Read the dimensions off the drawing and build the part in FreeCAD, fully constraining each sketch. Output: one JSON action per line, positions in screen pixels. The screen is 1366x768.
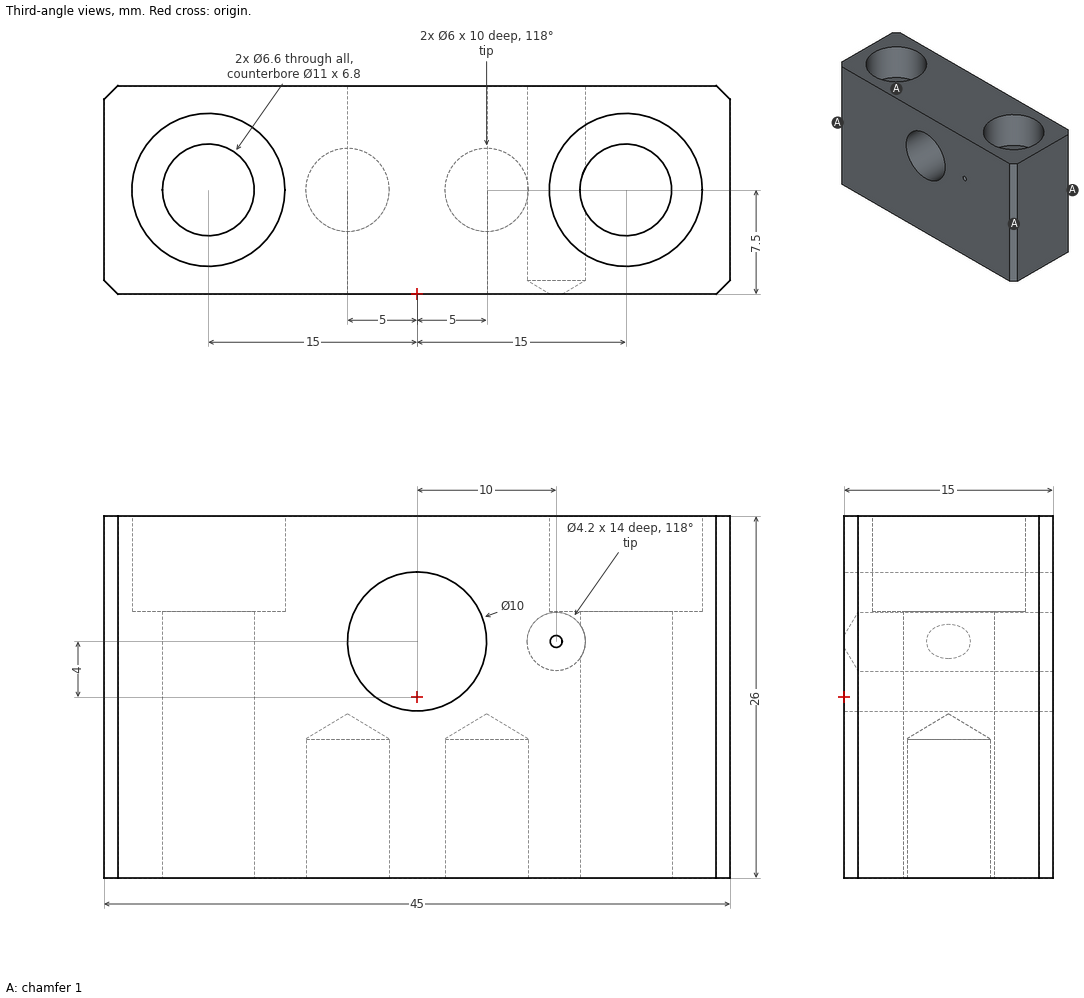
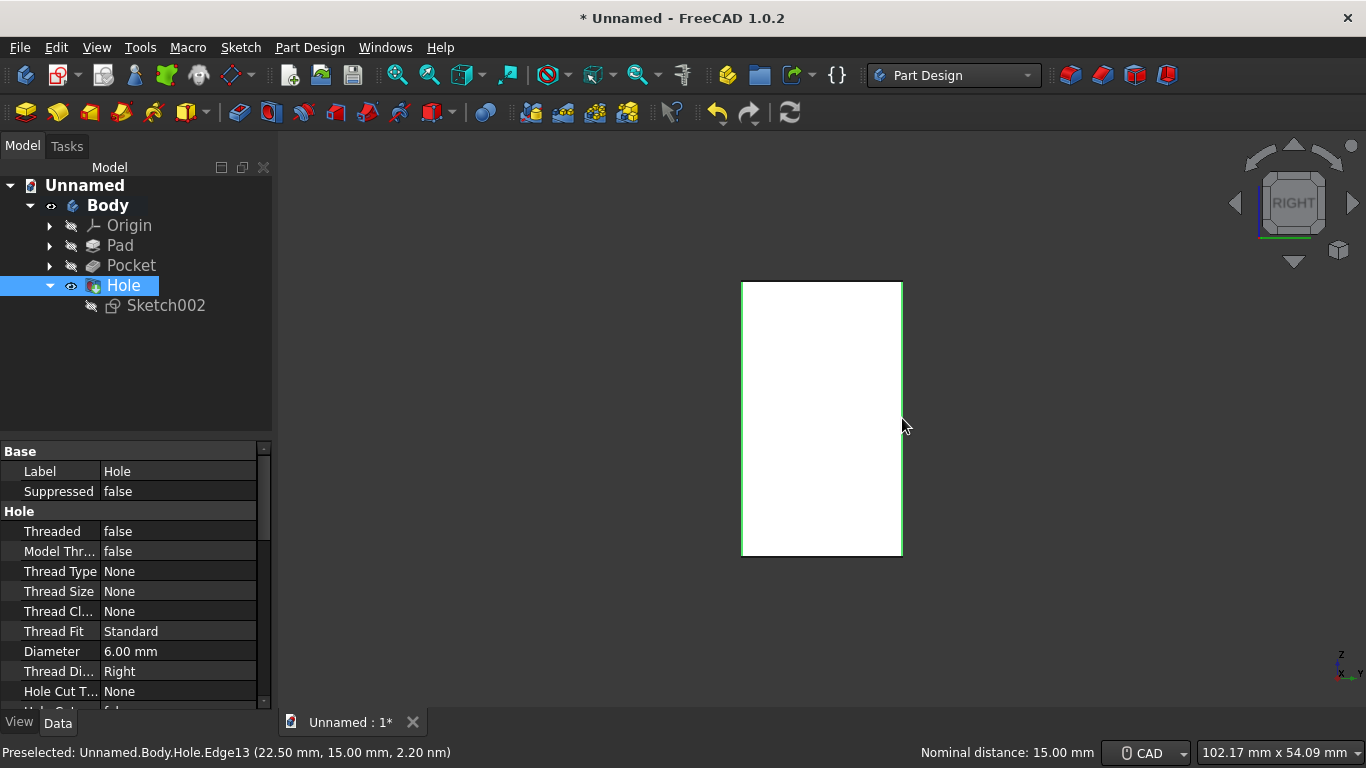
{"action": "key", "text": "5"}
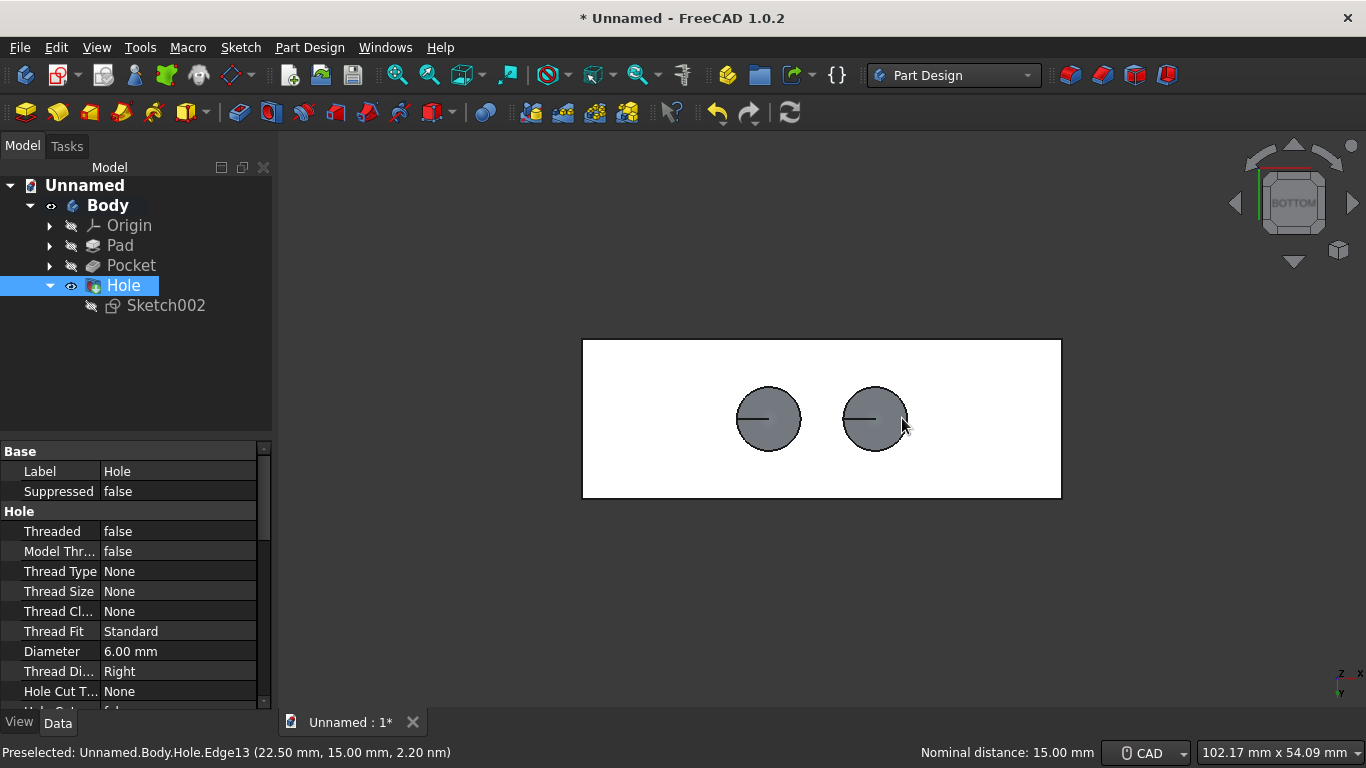
{"action": "left_click", "coordinate": [398, 76]}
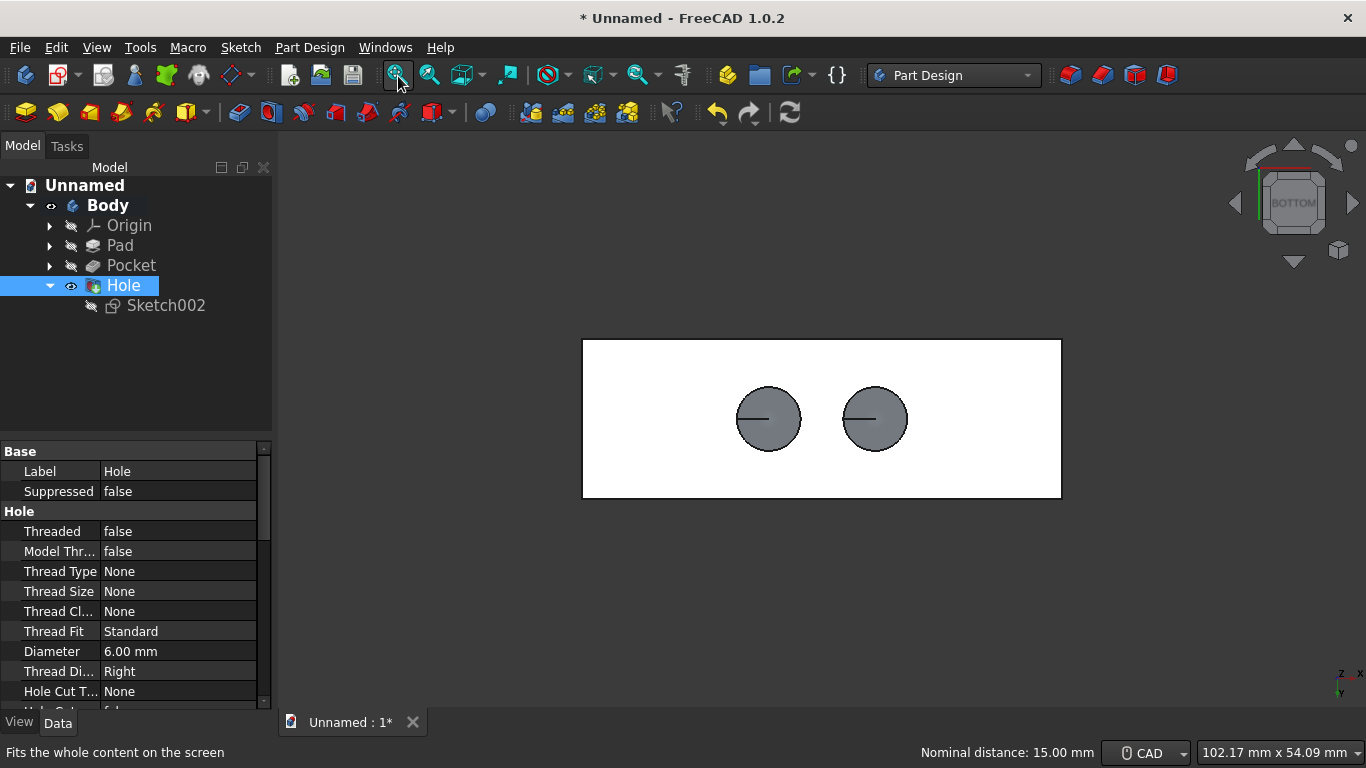
{"action": "key", "text": "4"}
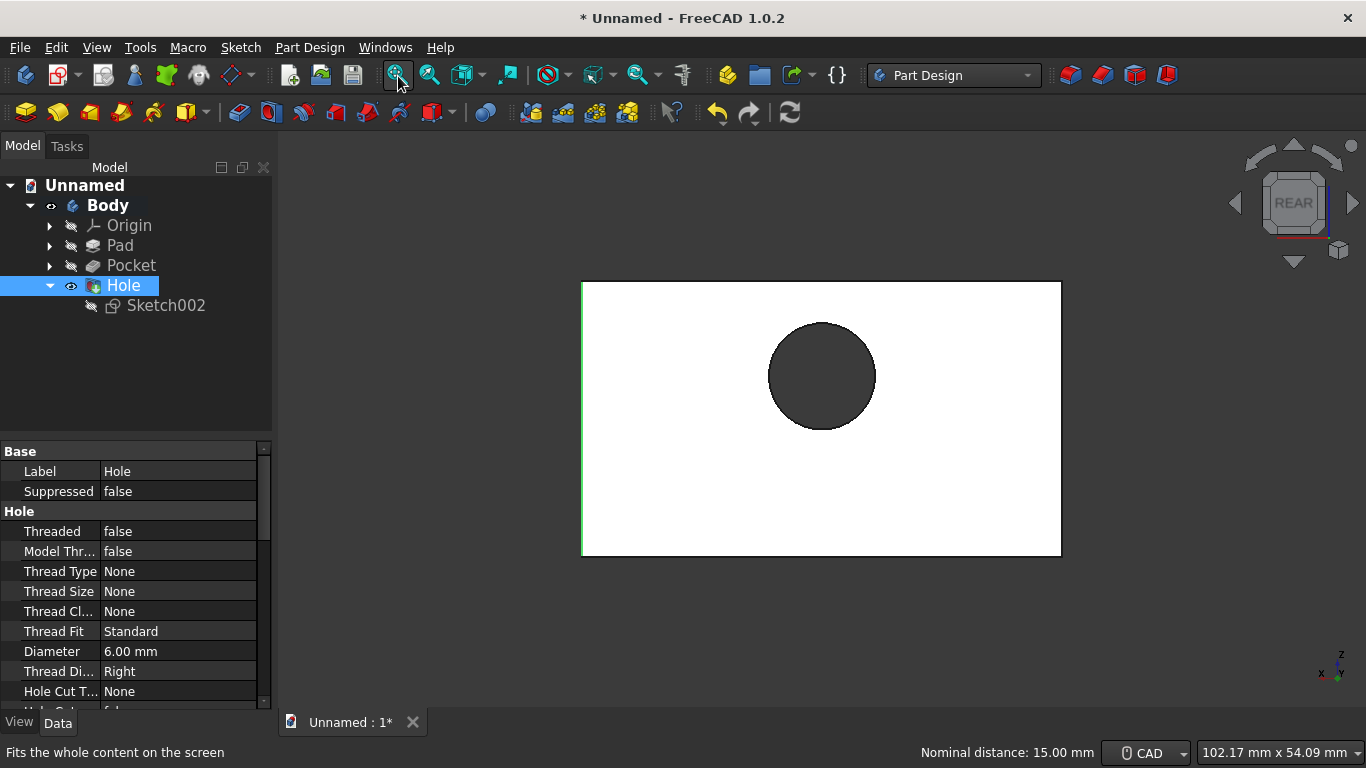
{"action": "left_click", "coordinate": [1062, 418], "text": "ctrl"}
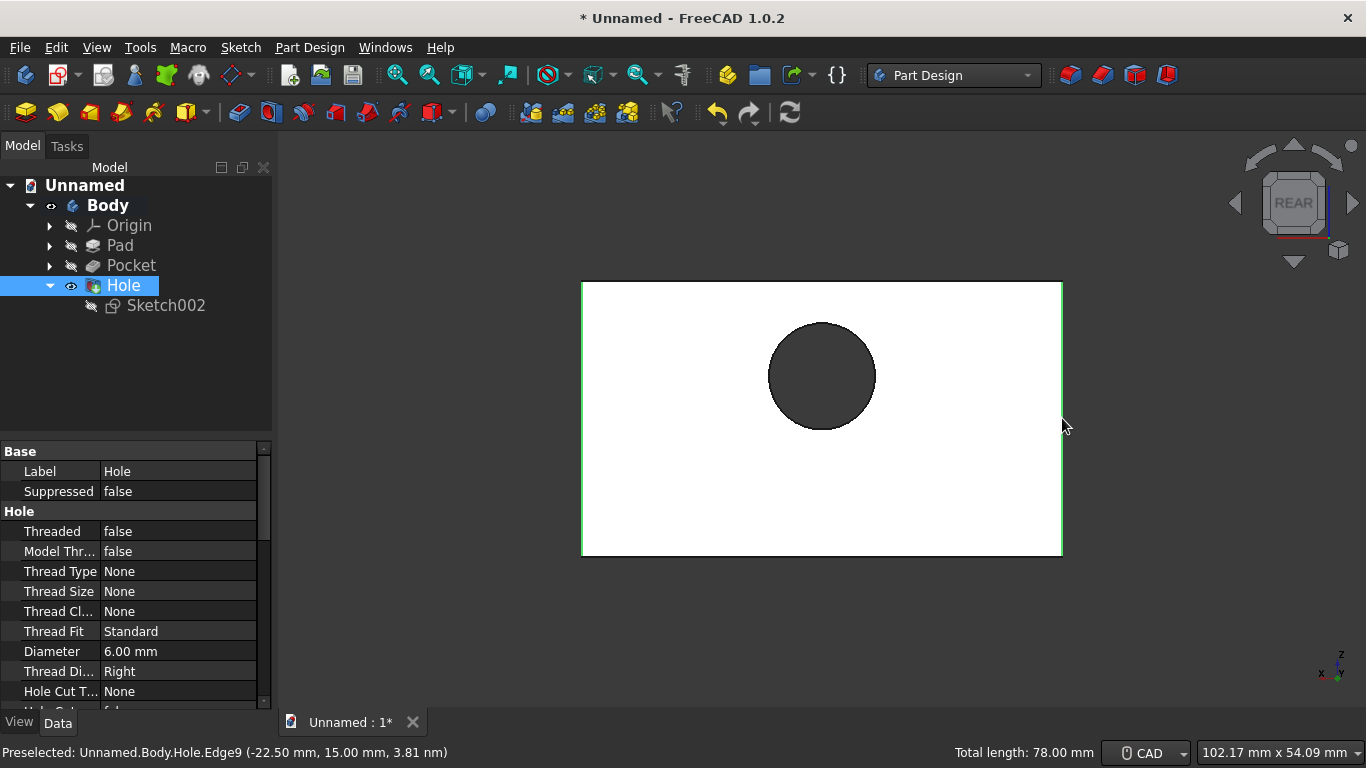
{"action": "key", "text": "6"}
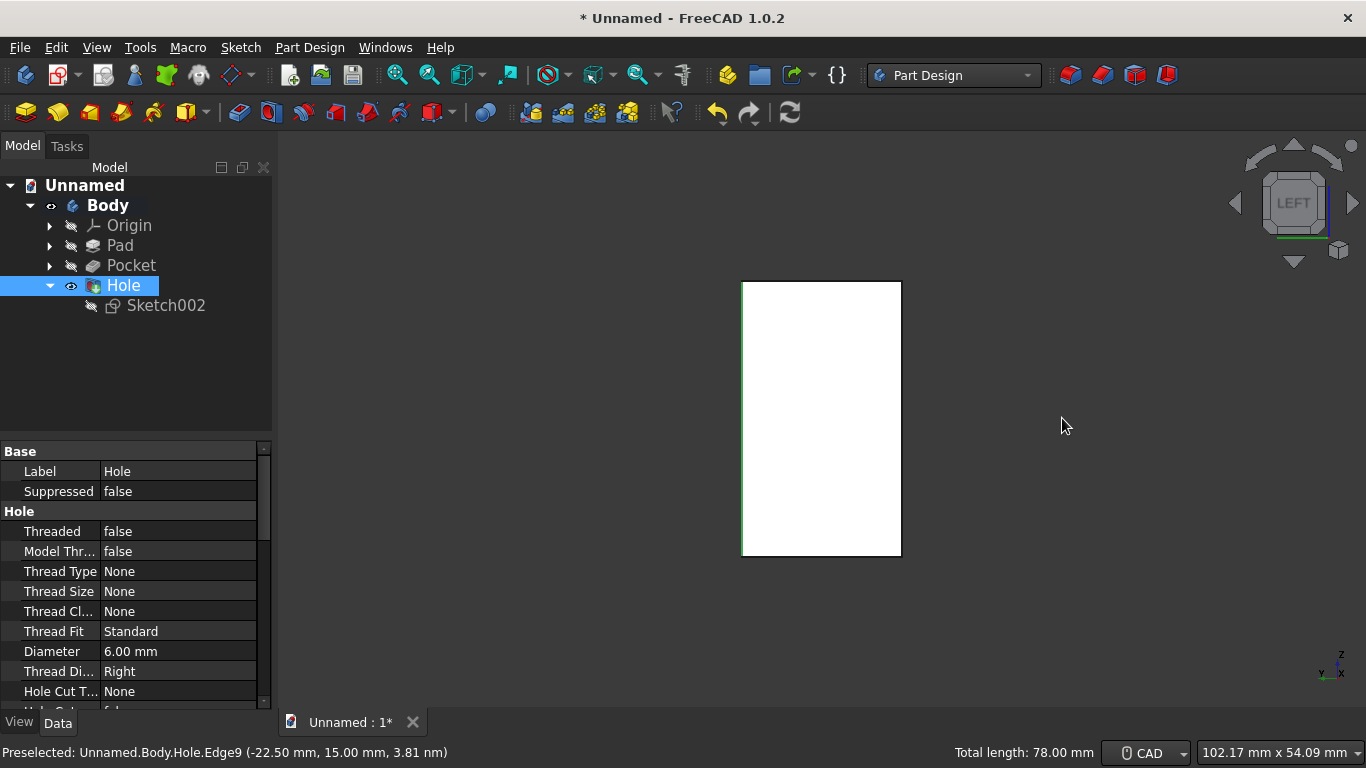
{"action": "left_click", "coordinate": [902, 418], "text": "ctrl"}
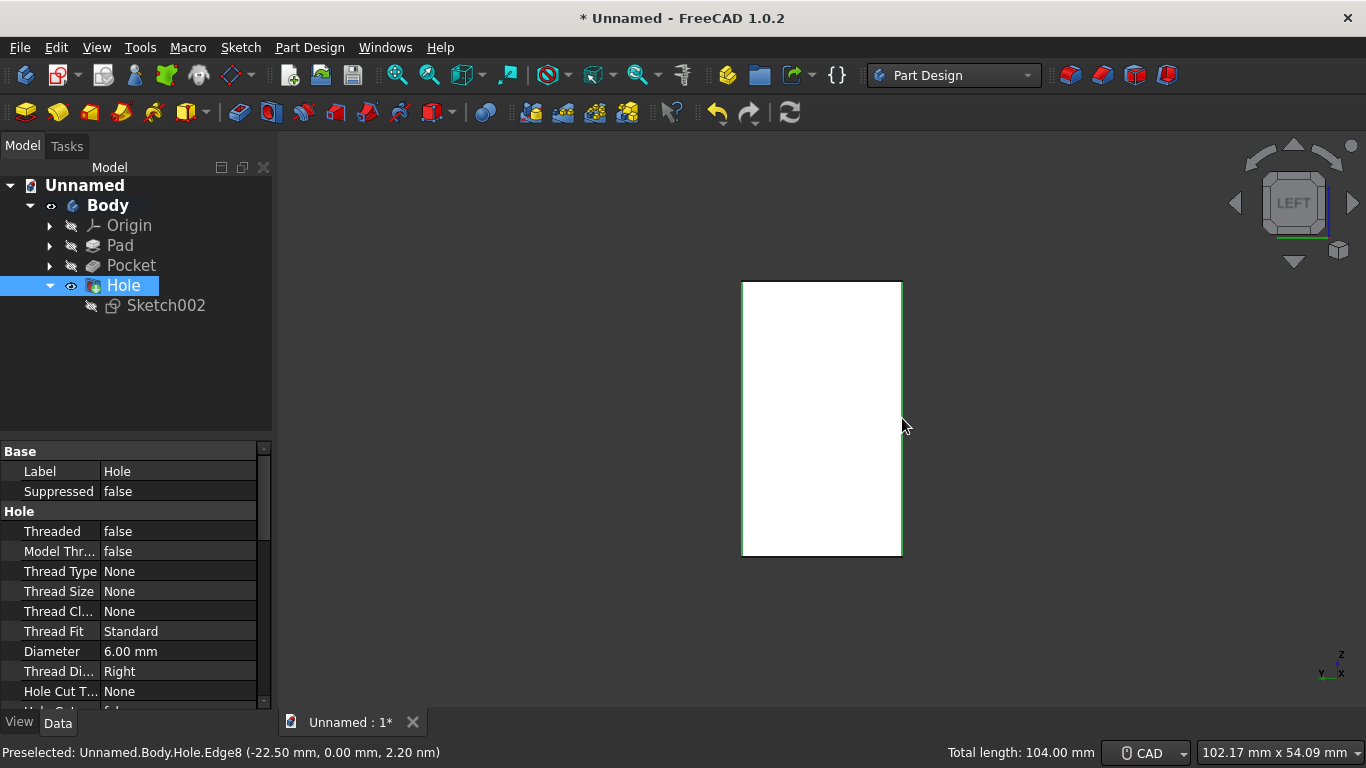
{"action": "left_click", "coordinate": [1104, 76]}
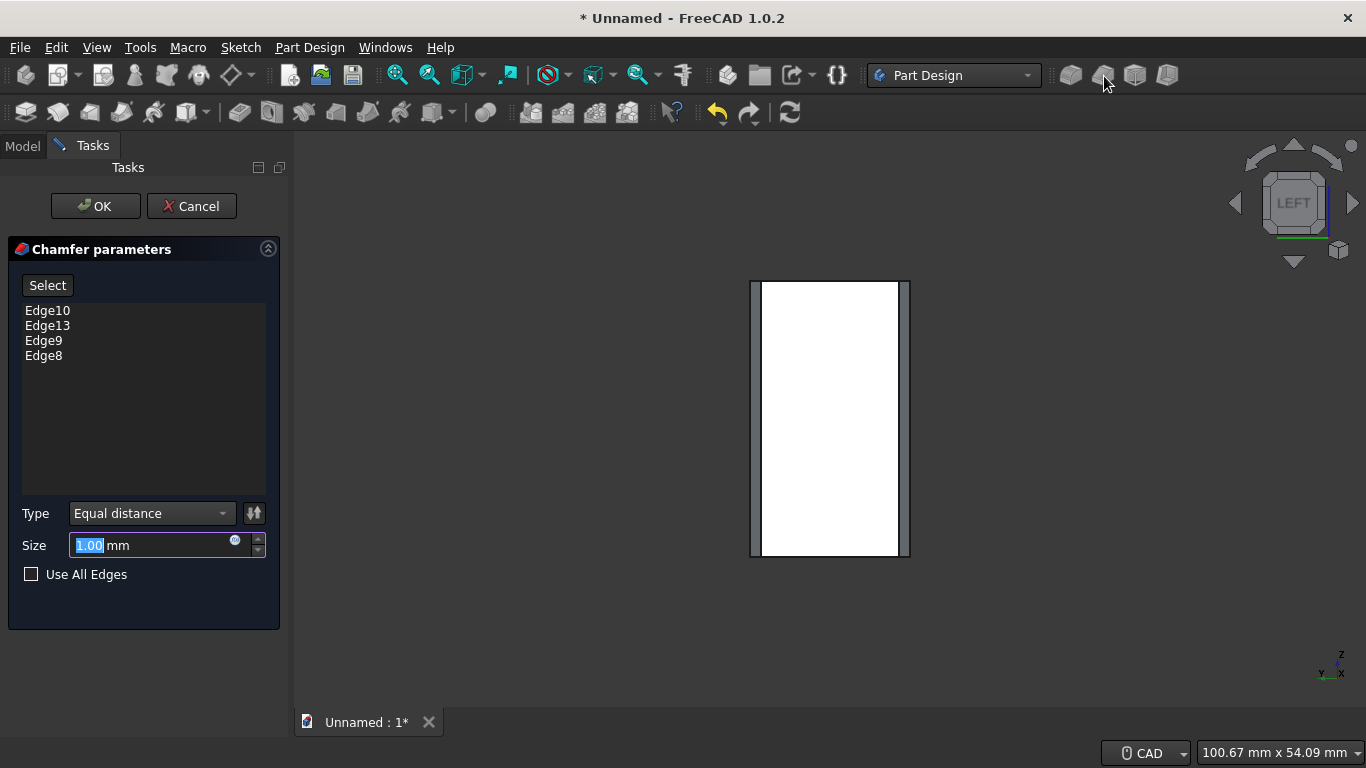
{"action": "type", "text": "1"}
{"action": "key", "text": "Tab"}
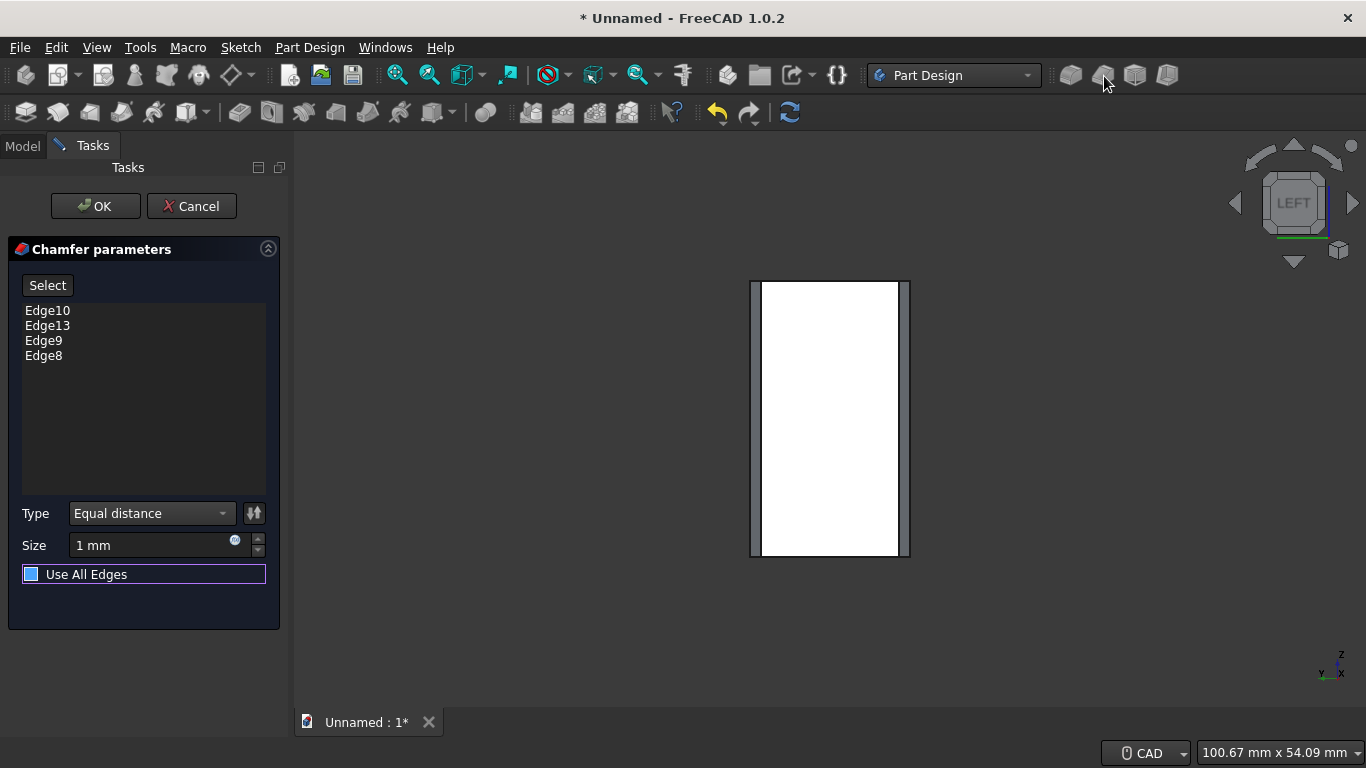
{"action": "left_click", "coordinate": [96, 206]}